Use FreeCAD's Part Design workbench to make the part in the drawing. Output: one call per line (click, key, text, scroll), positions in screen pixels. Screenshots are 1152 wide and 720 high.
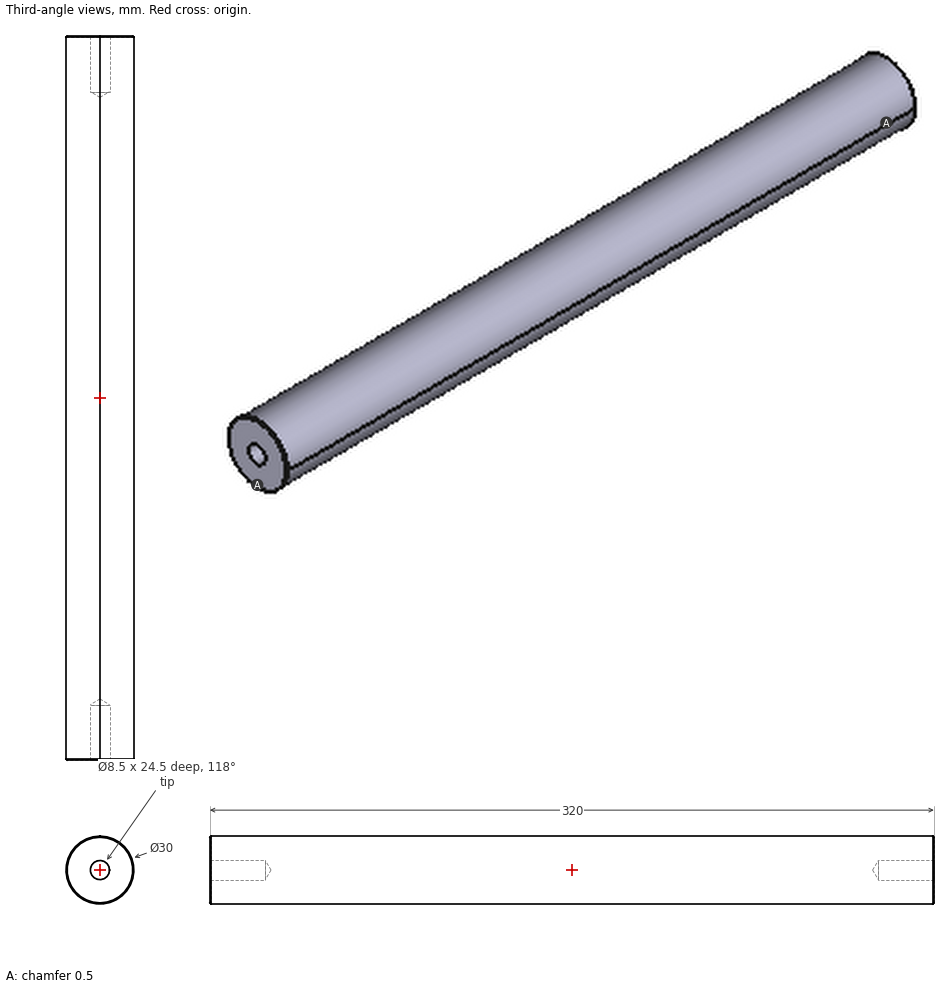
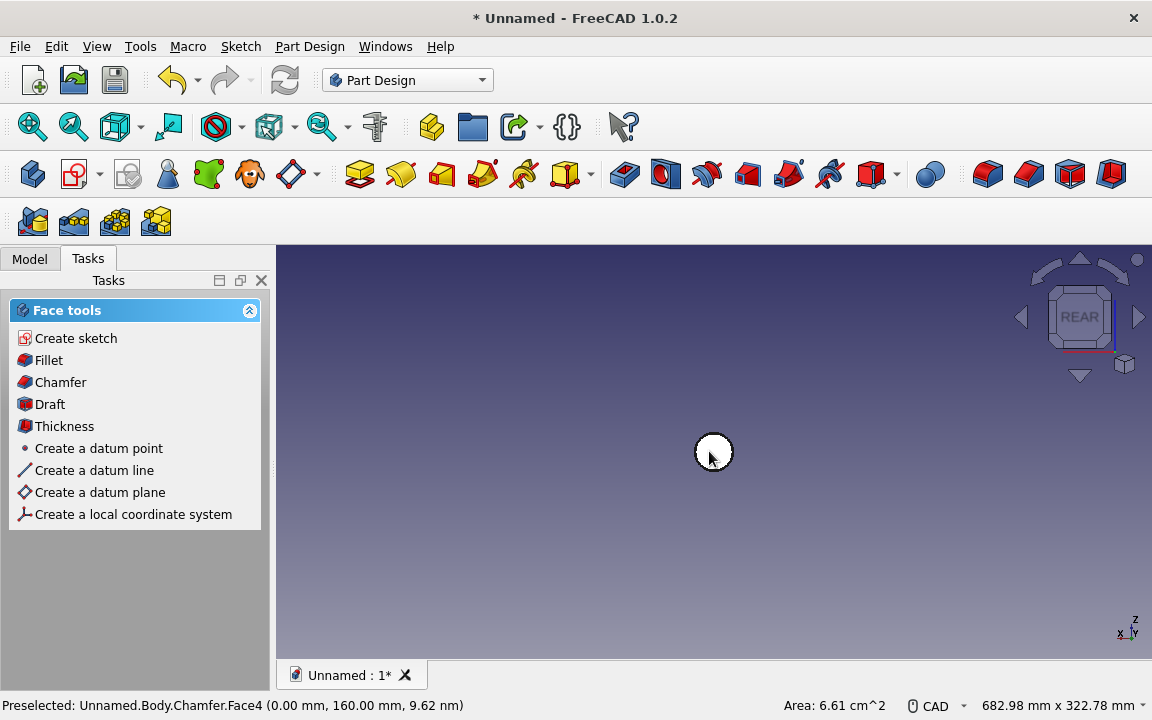
click(74, 174)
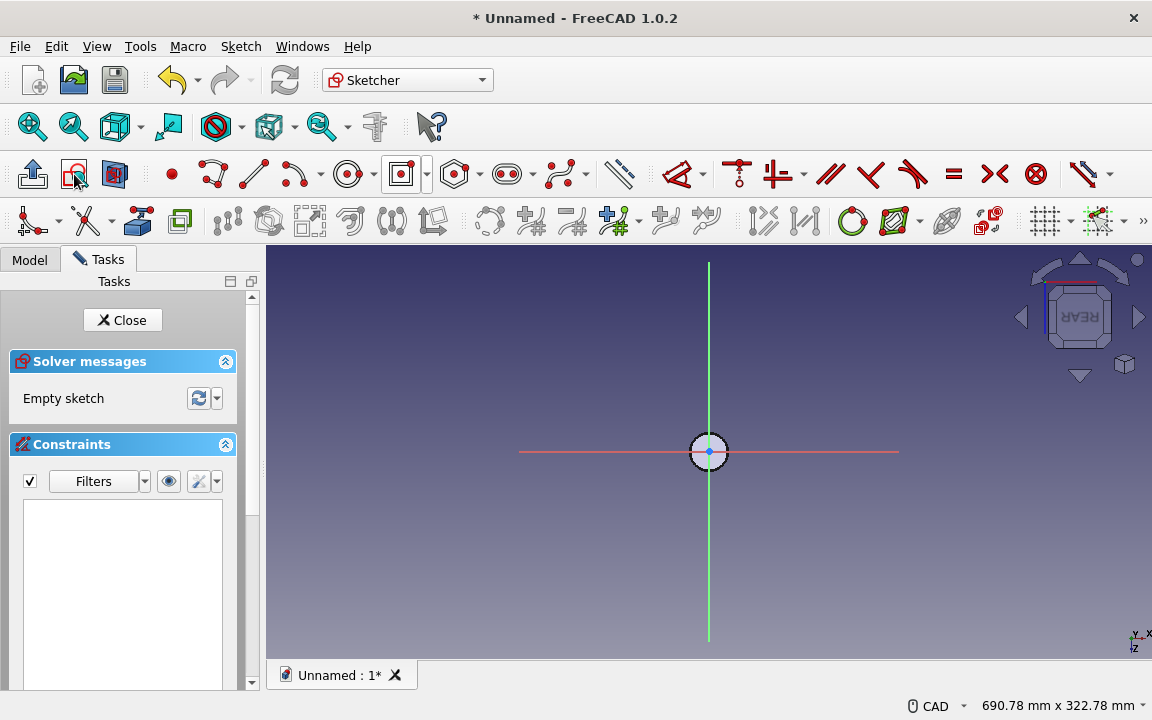
scroll(713, 452, up, 15)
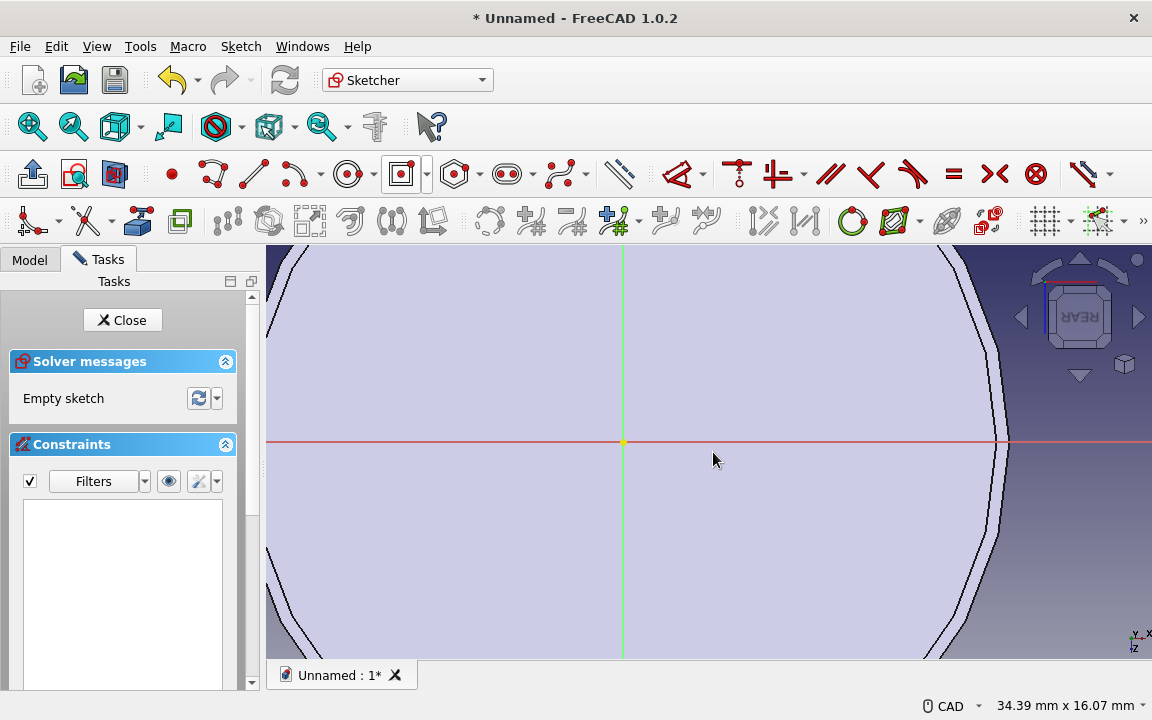
key(g)
key(c)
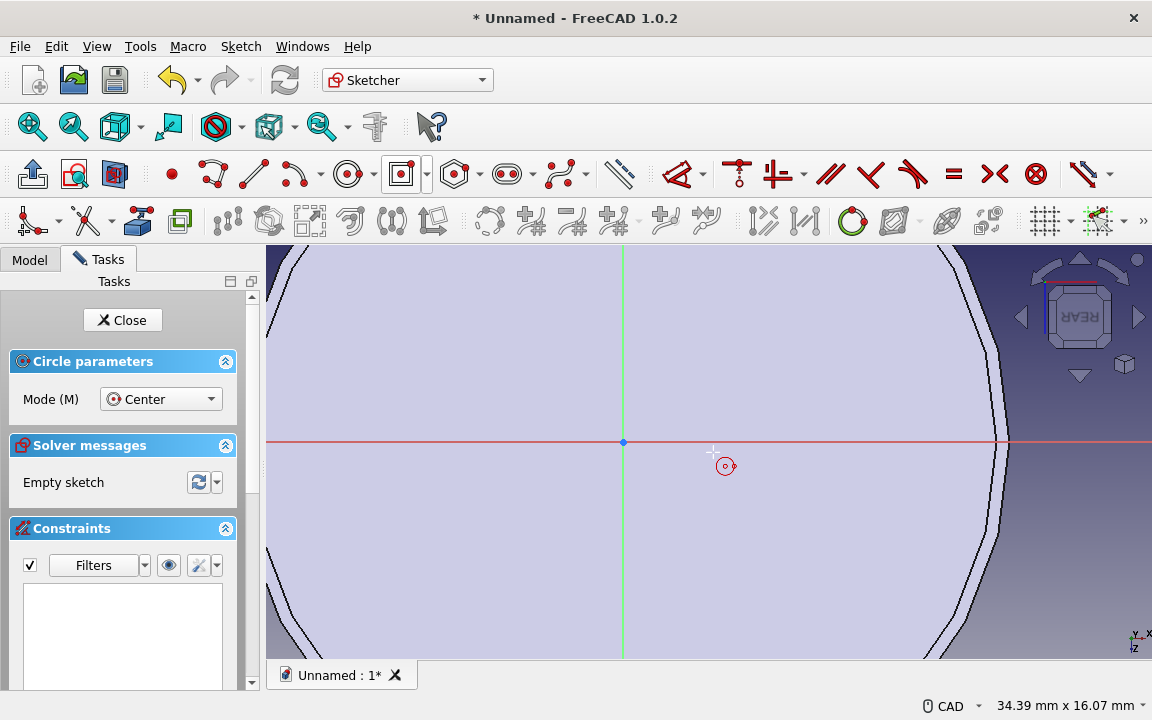
click(623, 442)
click(700, 365)
key(Escape)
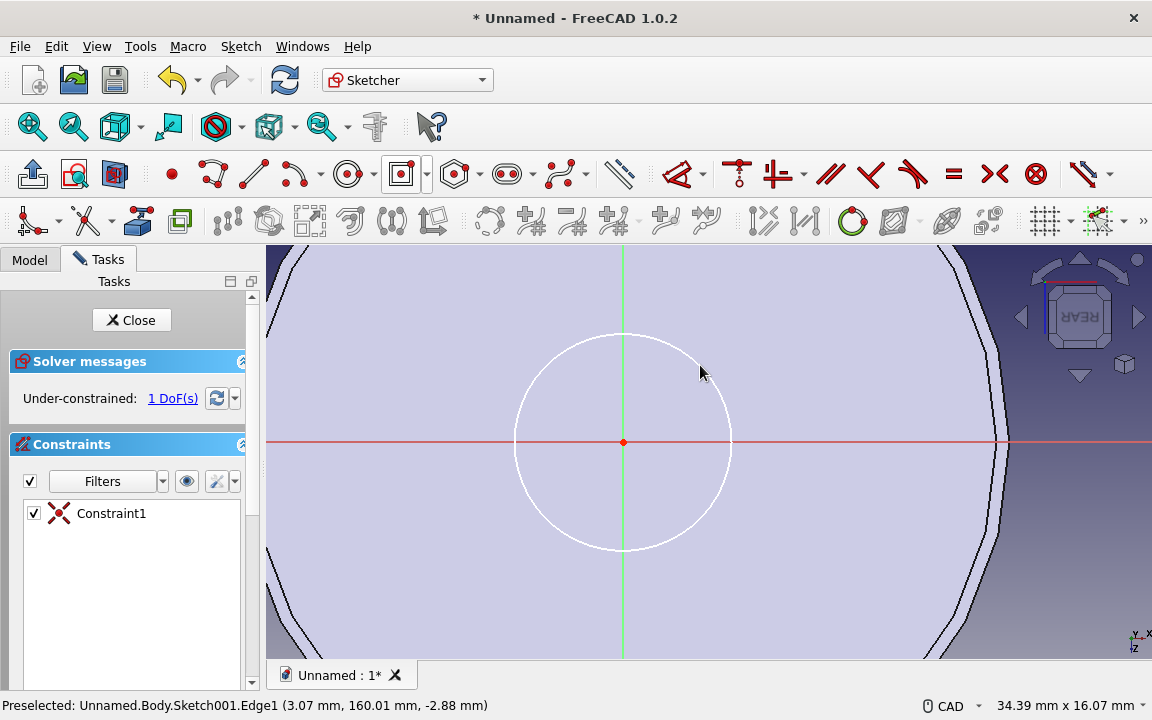
click(699, 365)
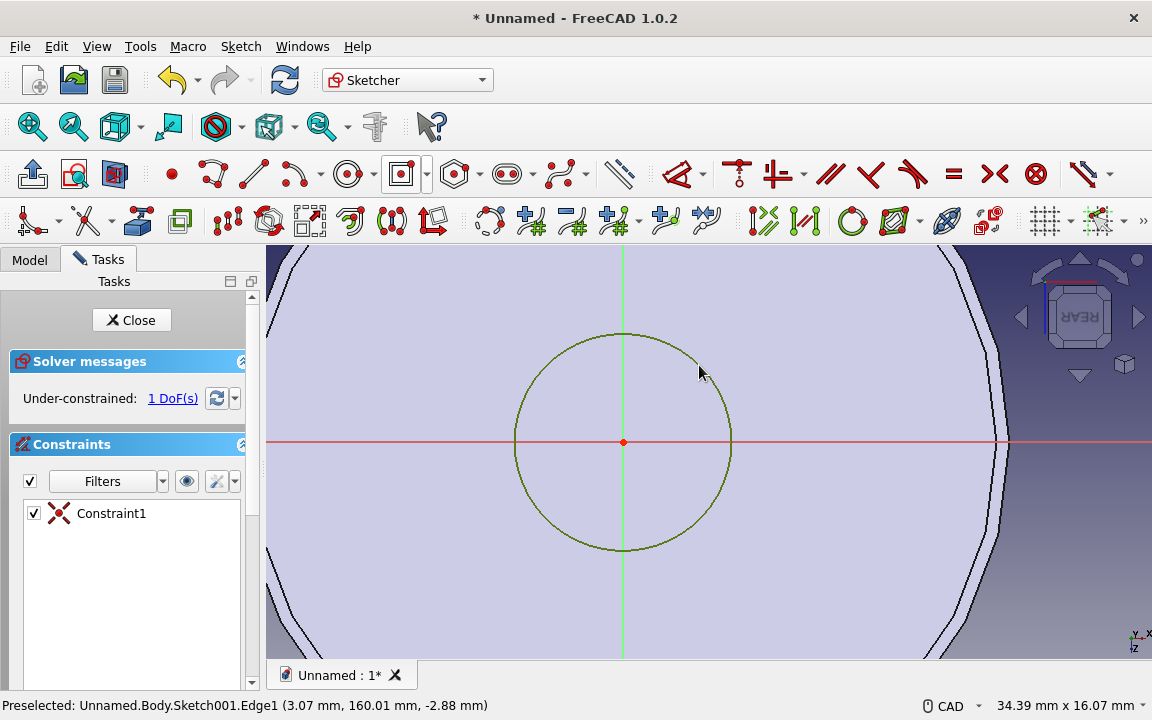
key(k)
key(o)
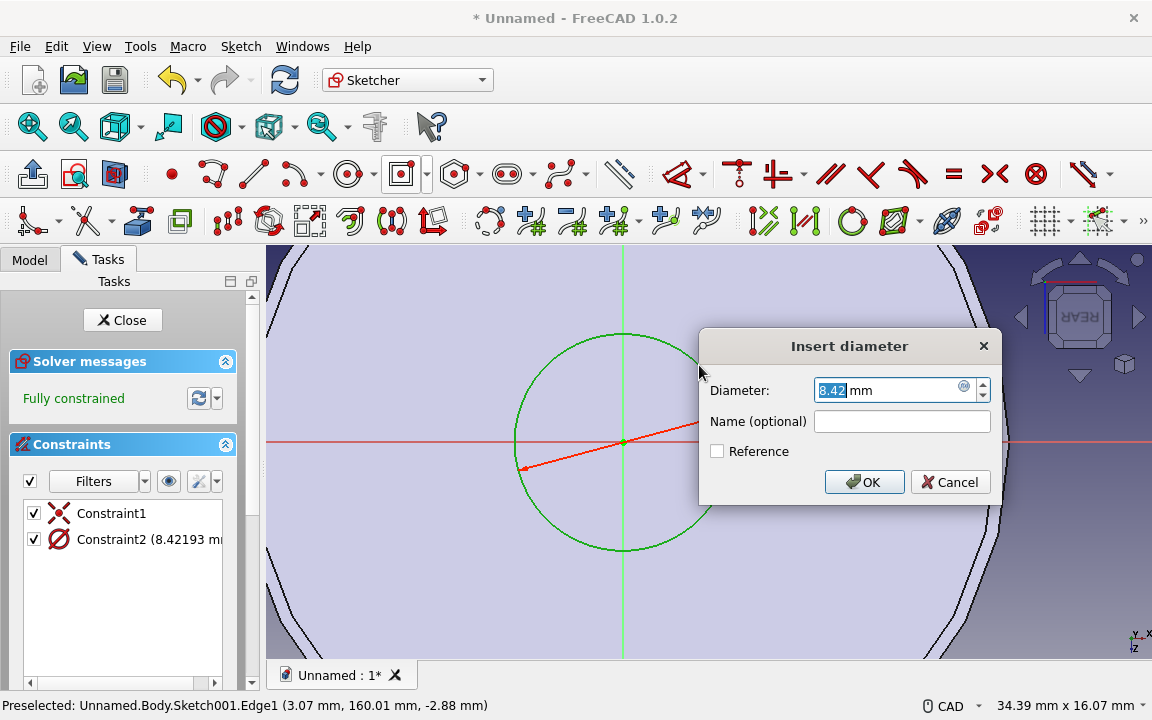
text(8.5)
key(Return)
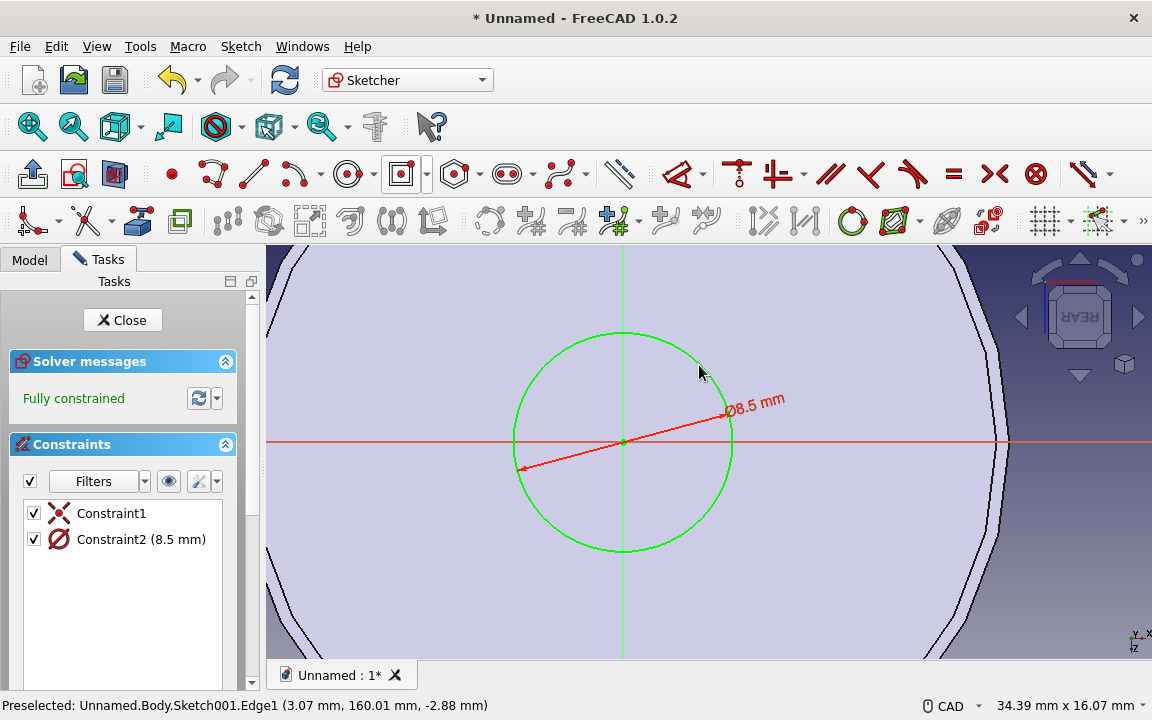
click(123, 320)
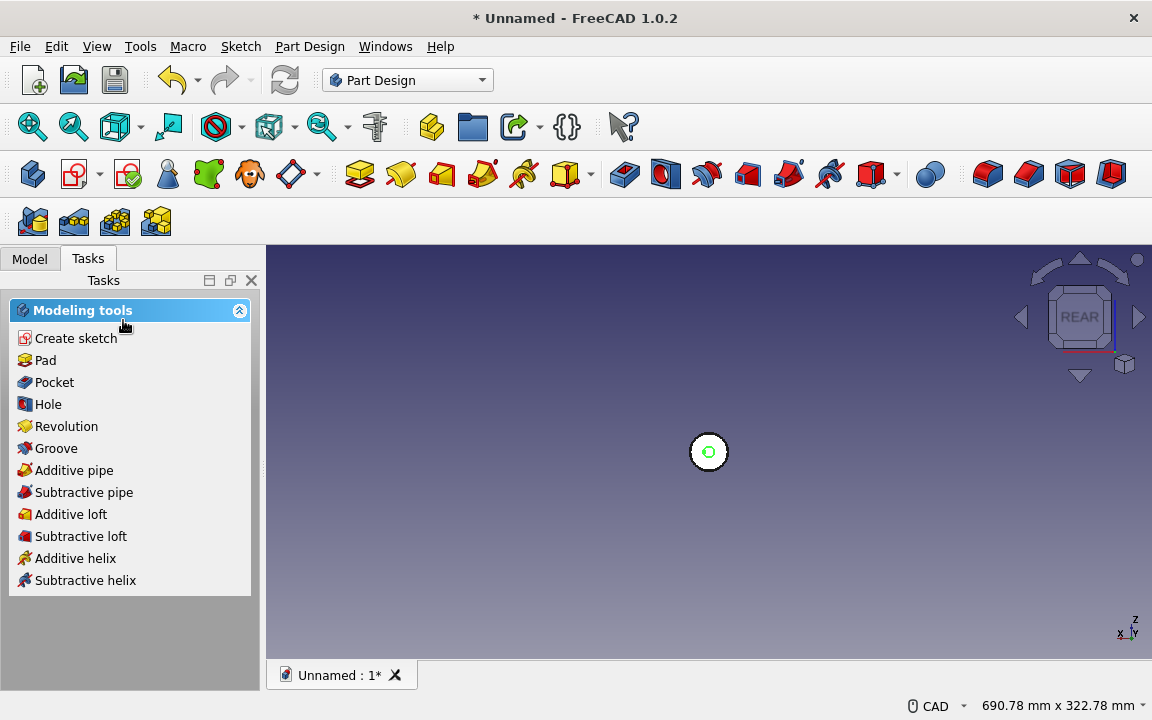
click(666, 174)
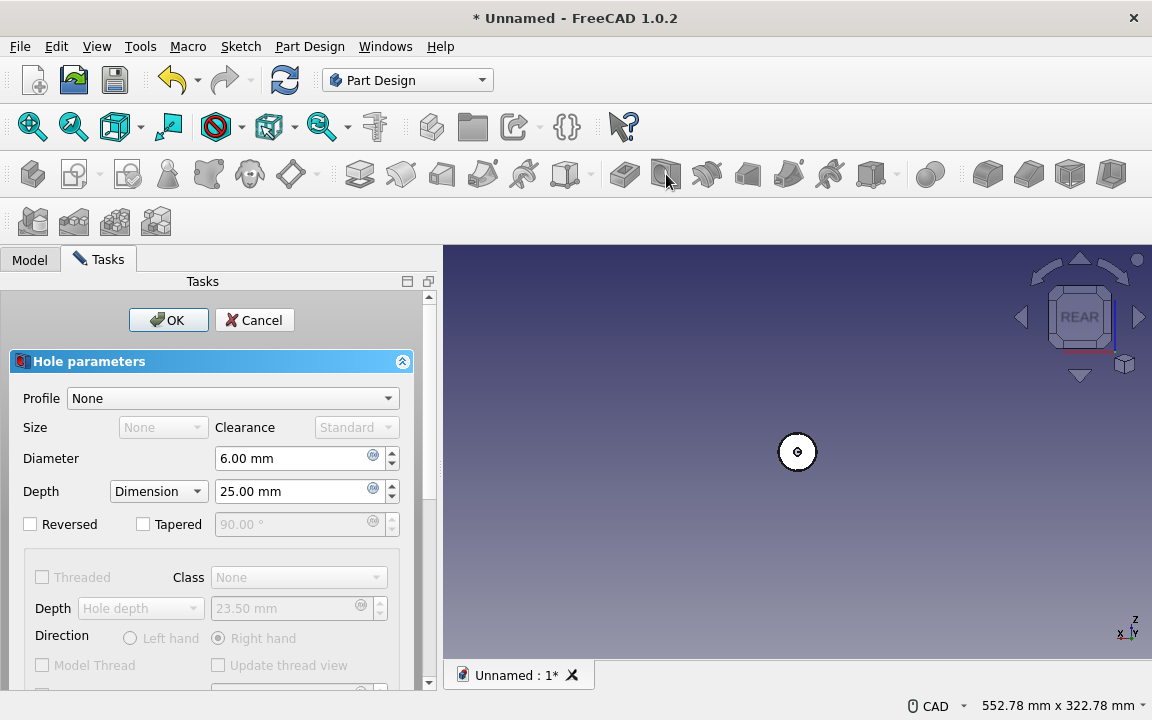
triple_click(300, 458)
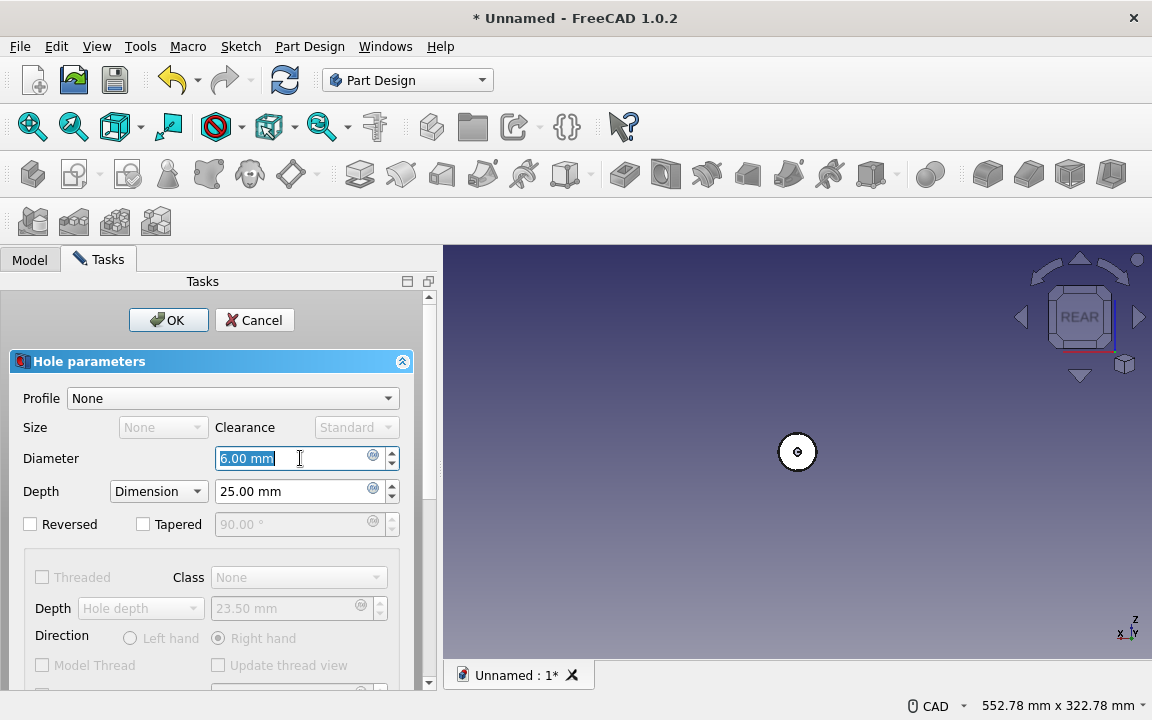
text(8.5)
key(Tab)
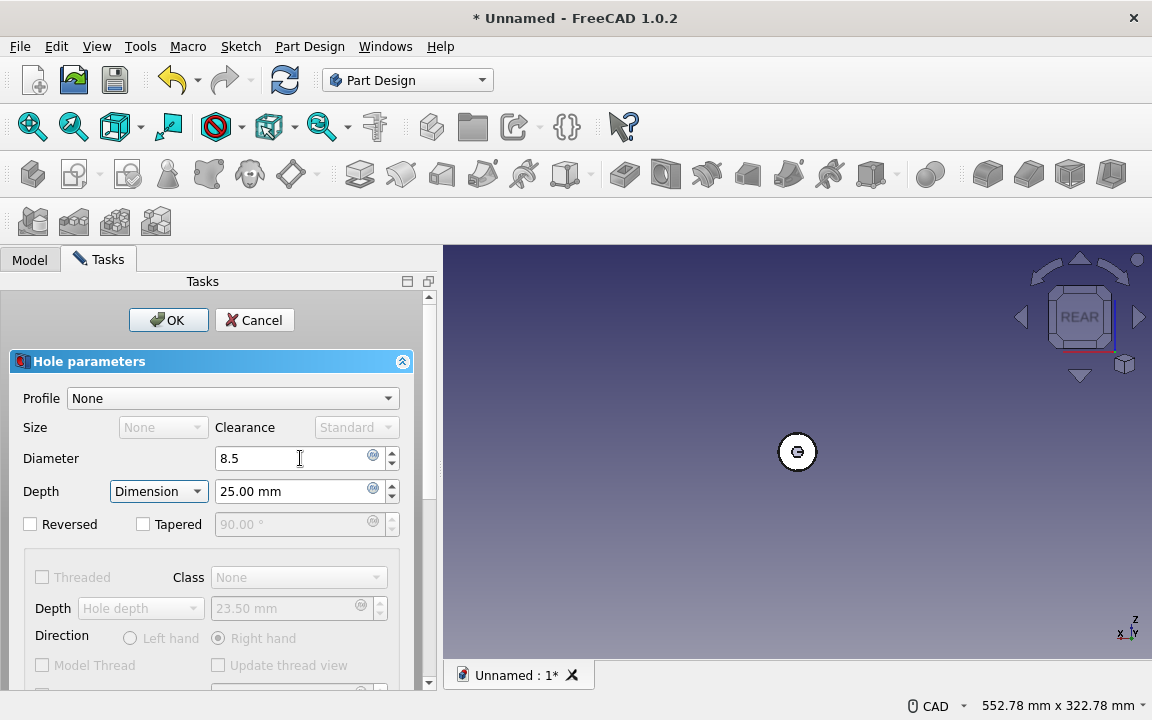
triple_click(300, 492)